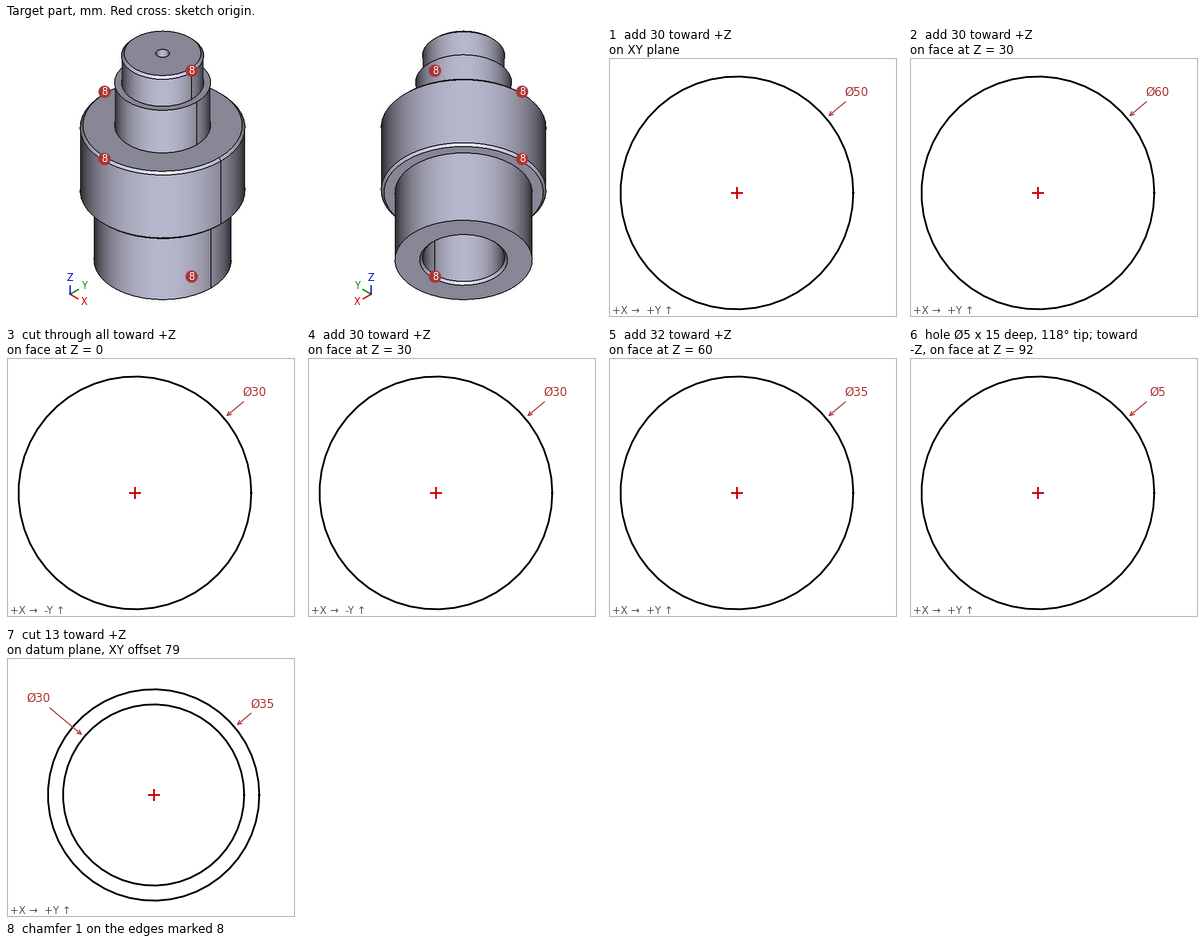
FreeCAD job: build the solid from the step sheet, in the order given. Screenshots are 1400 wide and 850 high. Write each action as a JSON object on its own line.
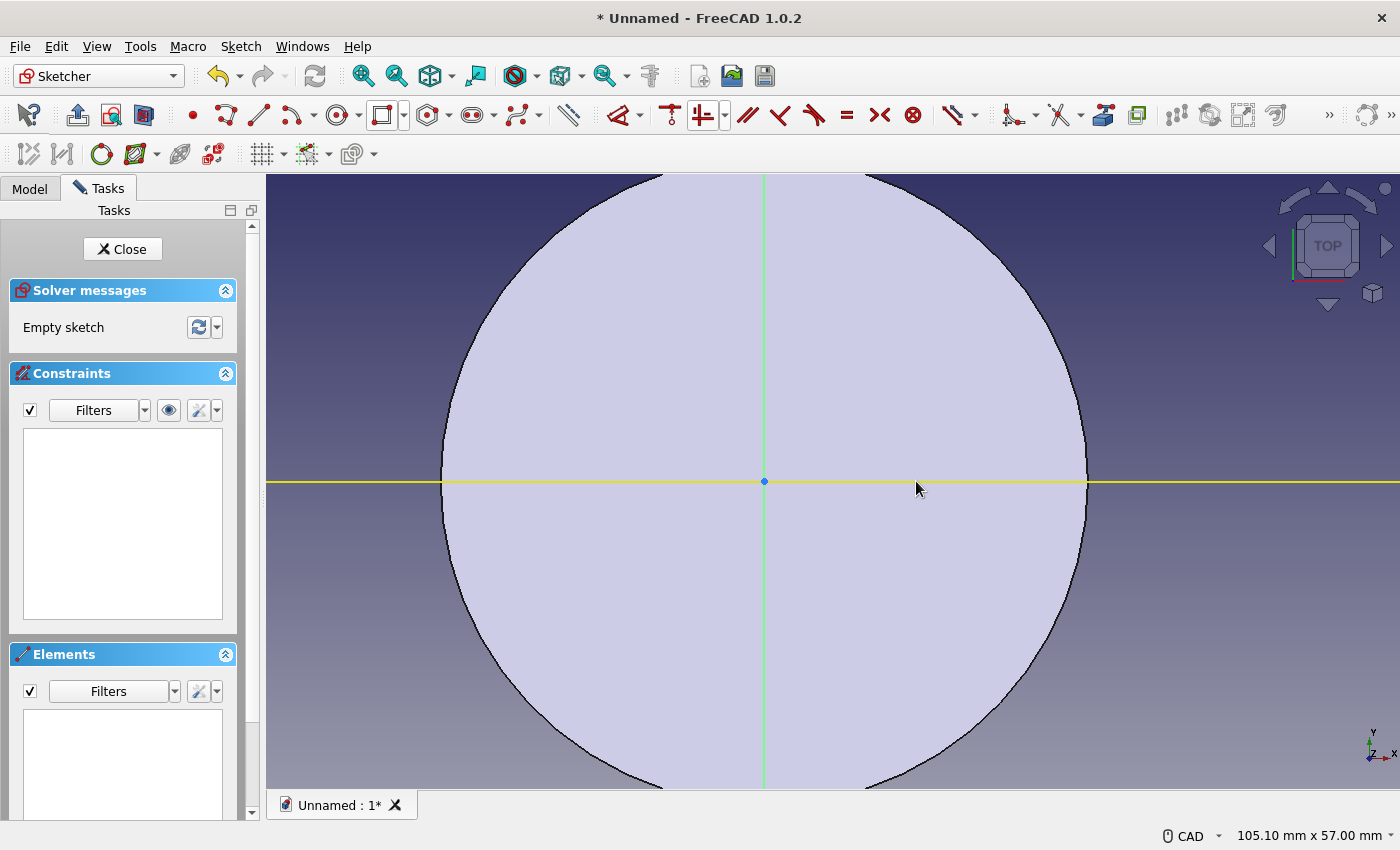
{"action": "left_click", "coordinate": [336, 116]}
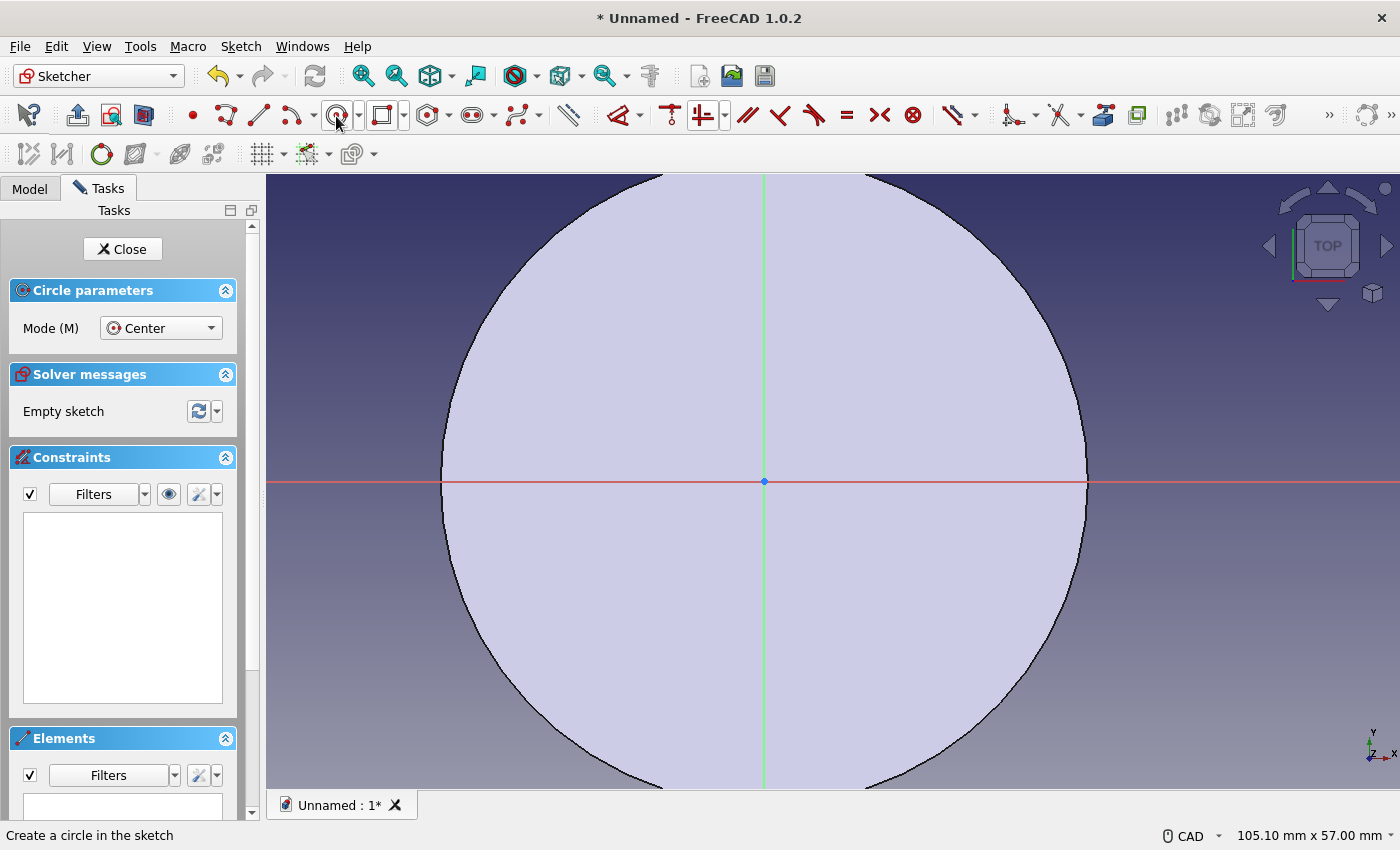
{"action": "left_click", "coordinate": [764, 482]}
{"action": "left_click", "coordinate": [898, 348]}
{"action": "key", "text": "Escape"}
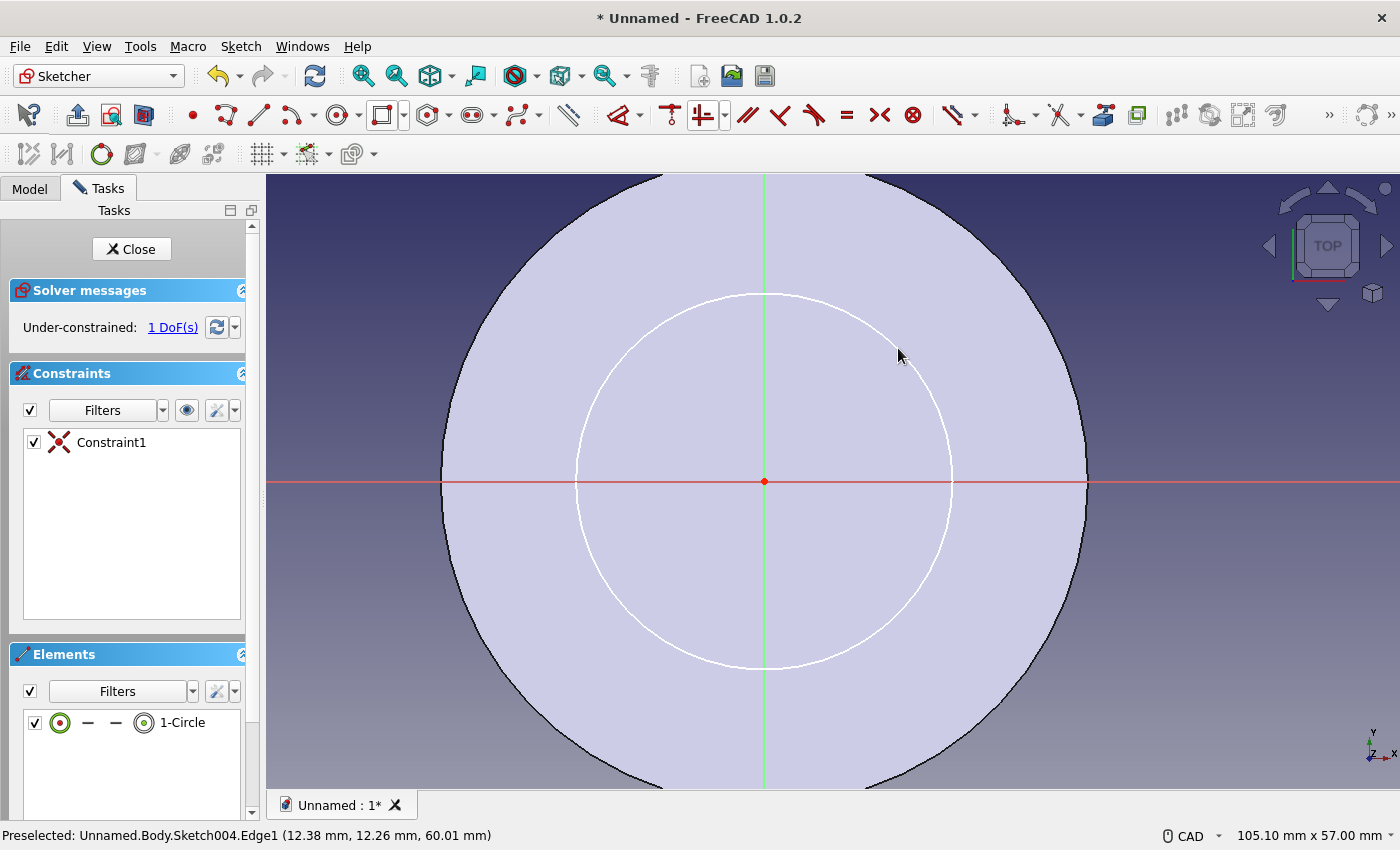
{"action": "key", "text": "d"}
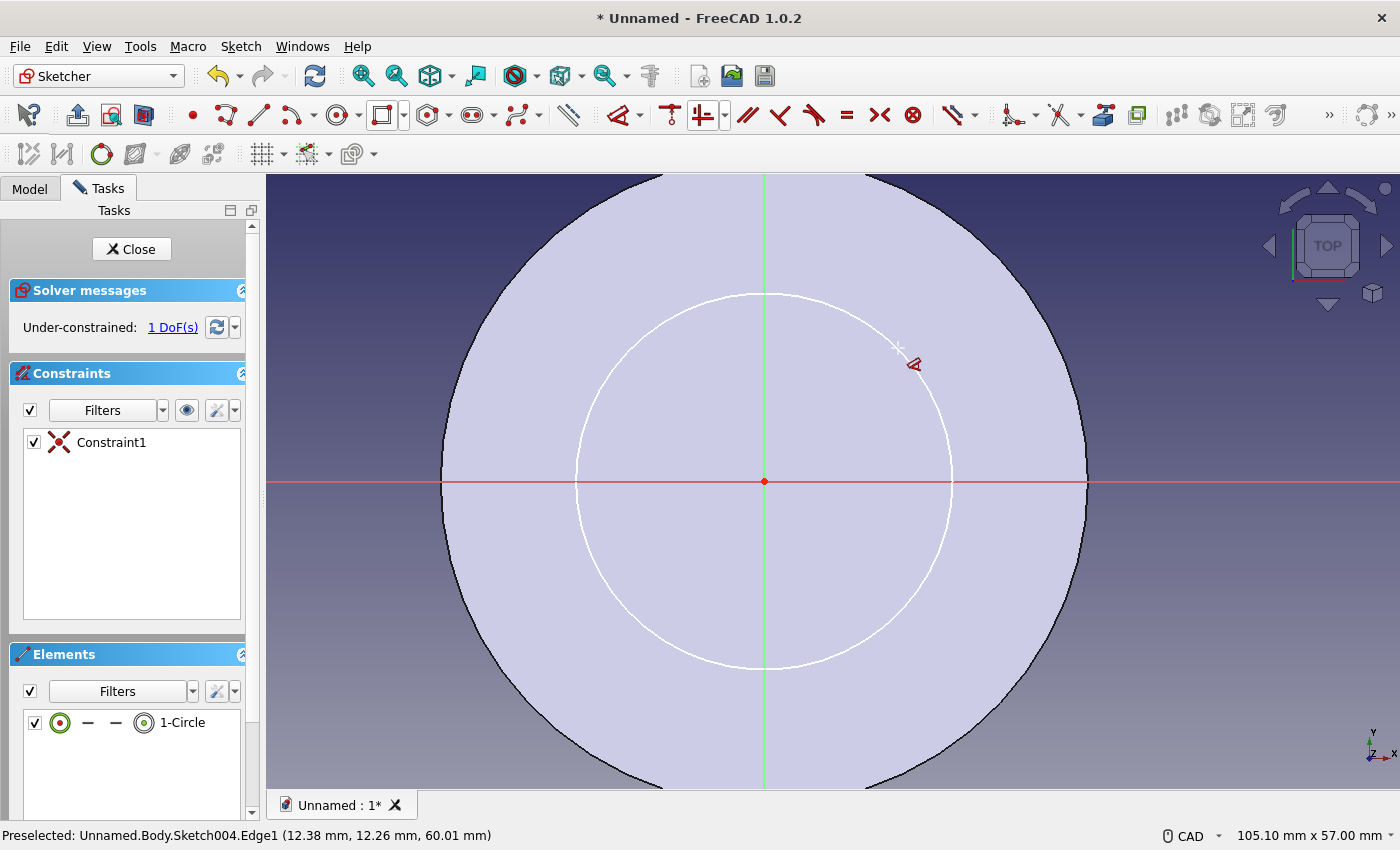
{"action": "left_click", "coordinate": [897, 348]}
{"action": "left_click", "coordinate": [920, 325]}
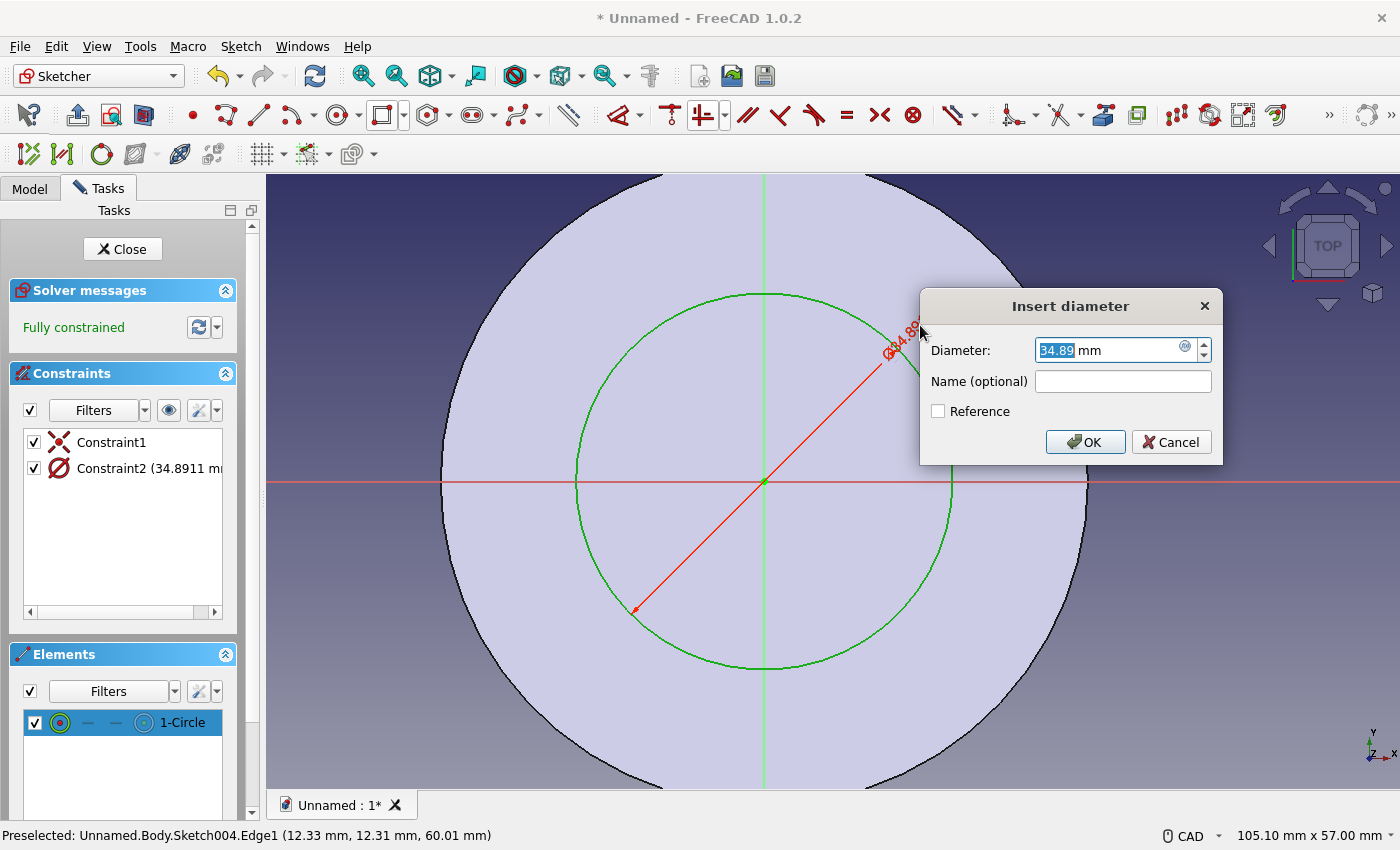
{"action": "type", "text": "35"}
{"action": "key", "text": "Return"}
{"action": "key", "text": "Escape"}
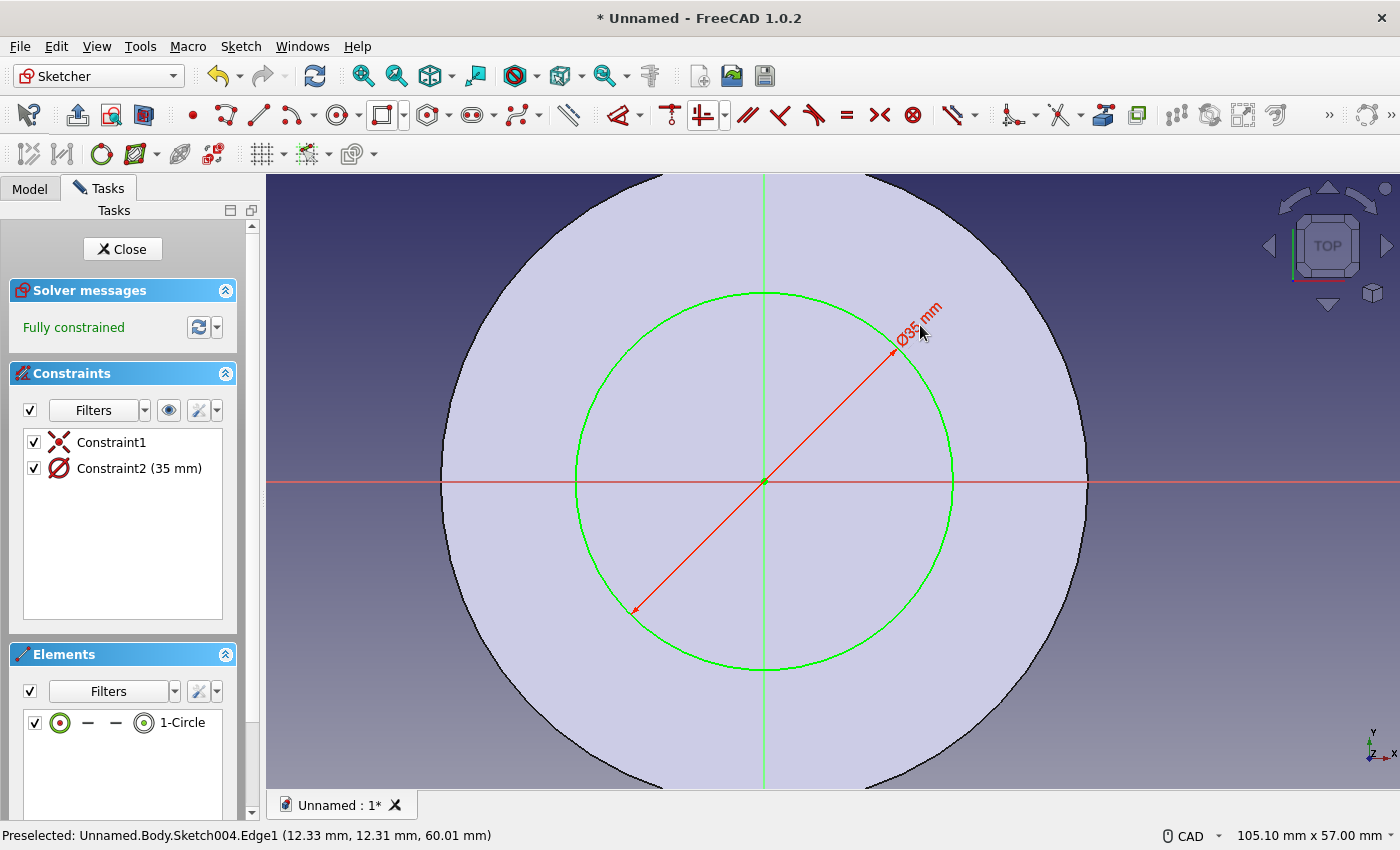
{"action": "left_click", "coordinate": [123, 249]}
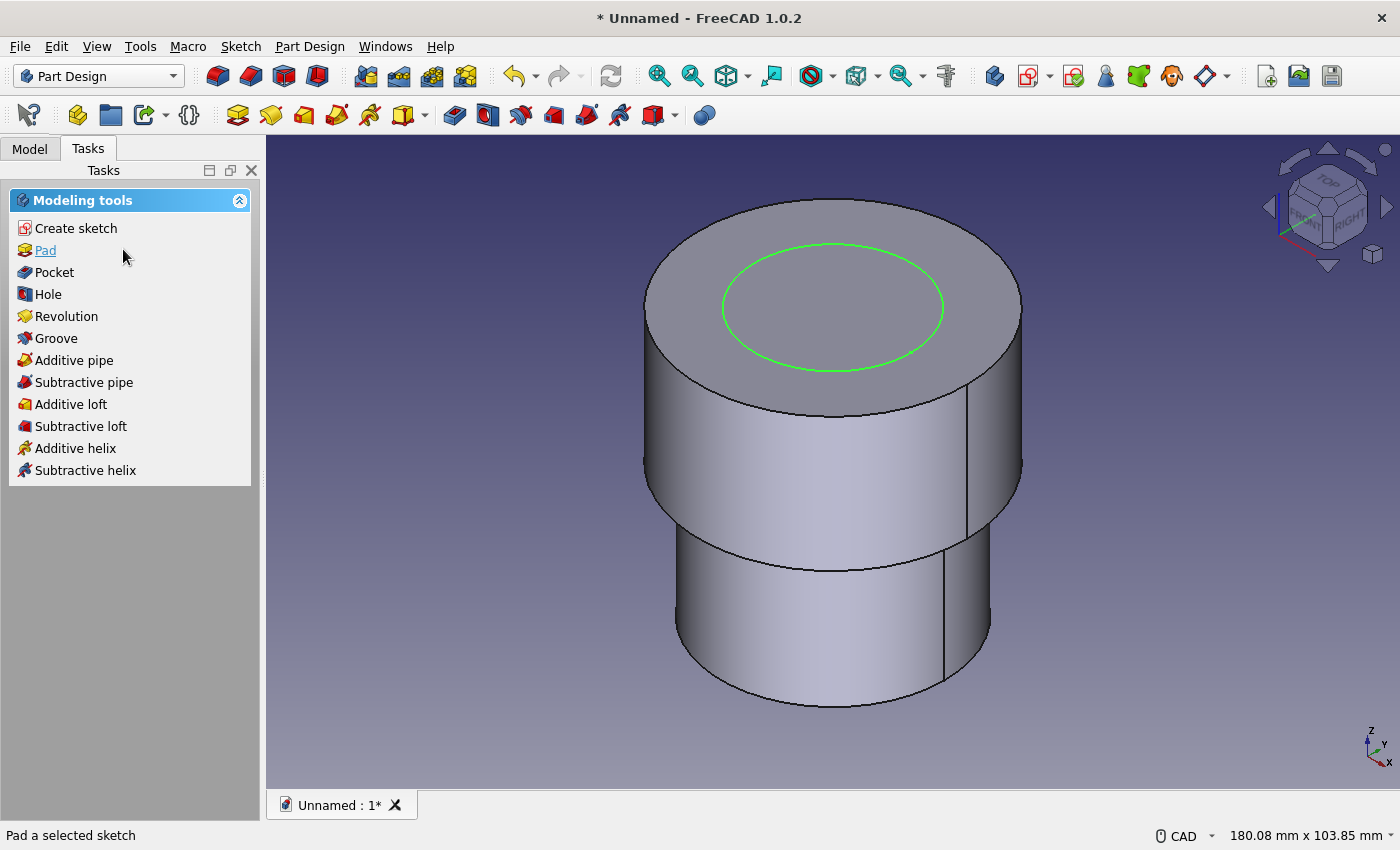
{"action": "left_click", "coordinate": [238, 116]}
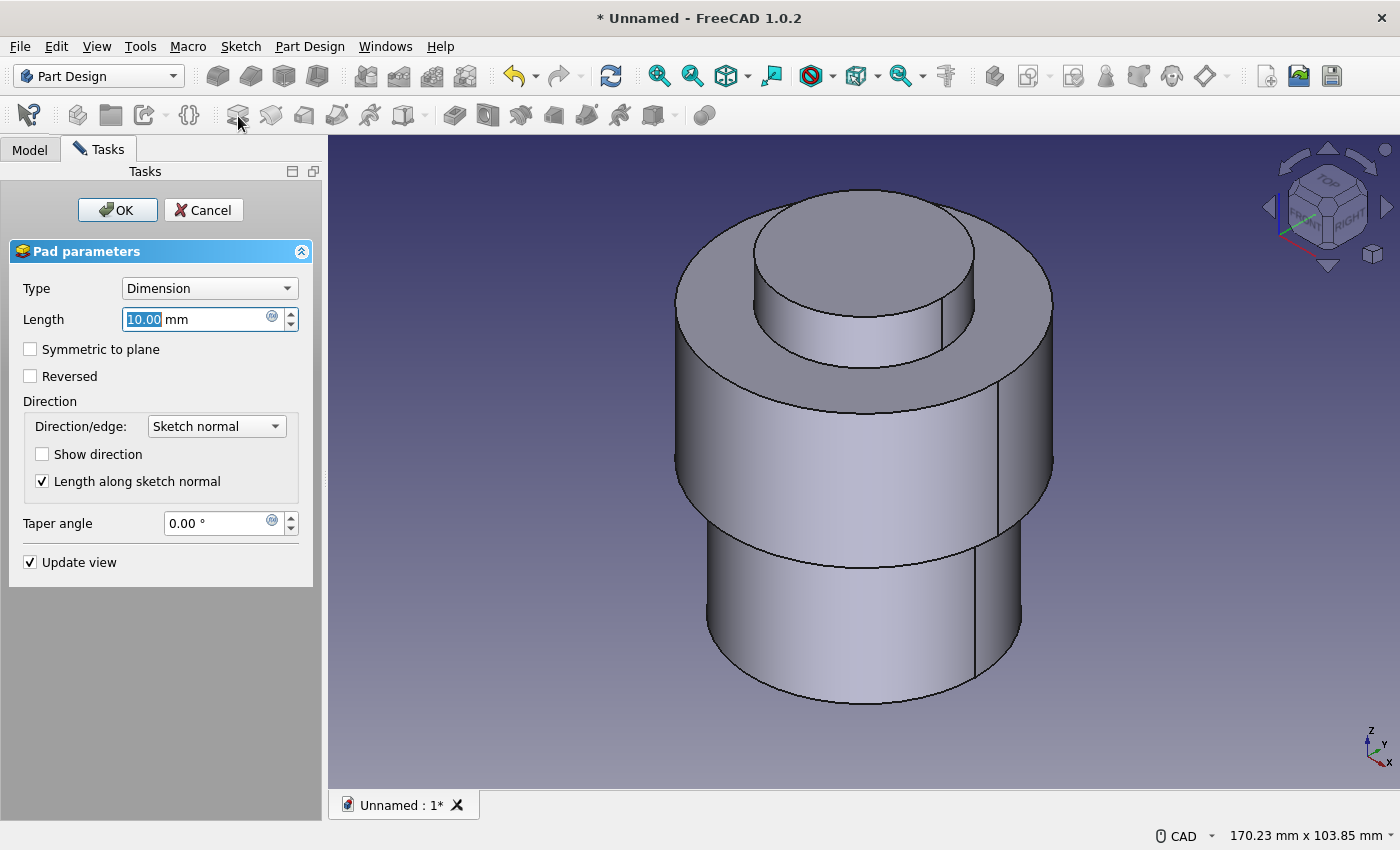
{"action": "type", "text": "32"}
{"action": "key", "text": "Tab"}